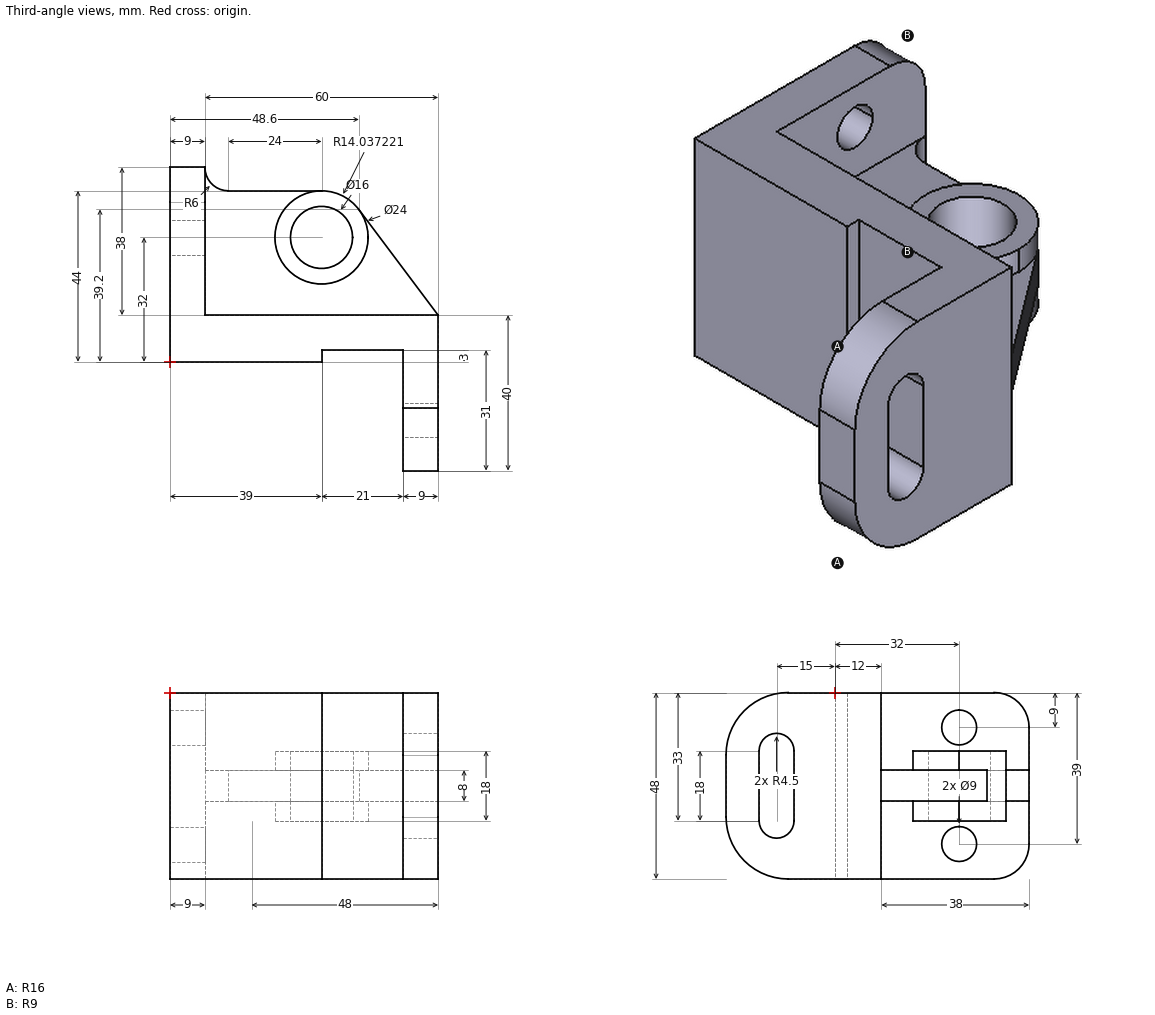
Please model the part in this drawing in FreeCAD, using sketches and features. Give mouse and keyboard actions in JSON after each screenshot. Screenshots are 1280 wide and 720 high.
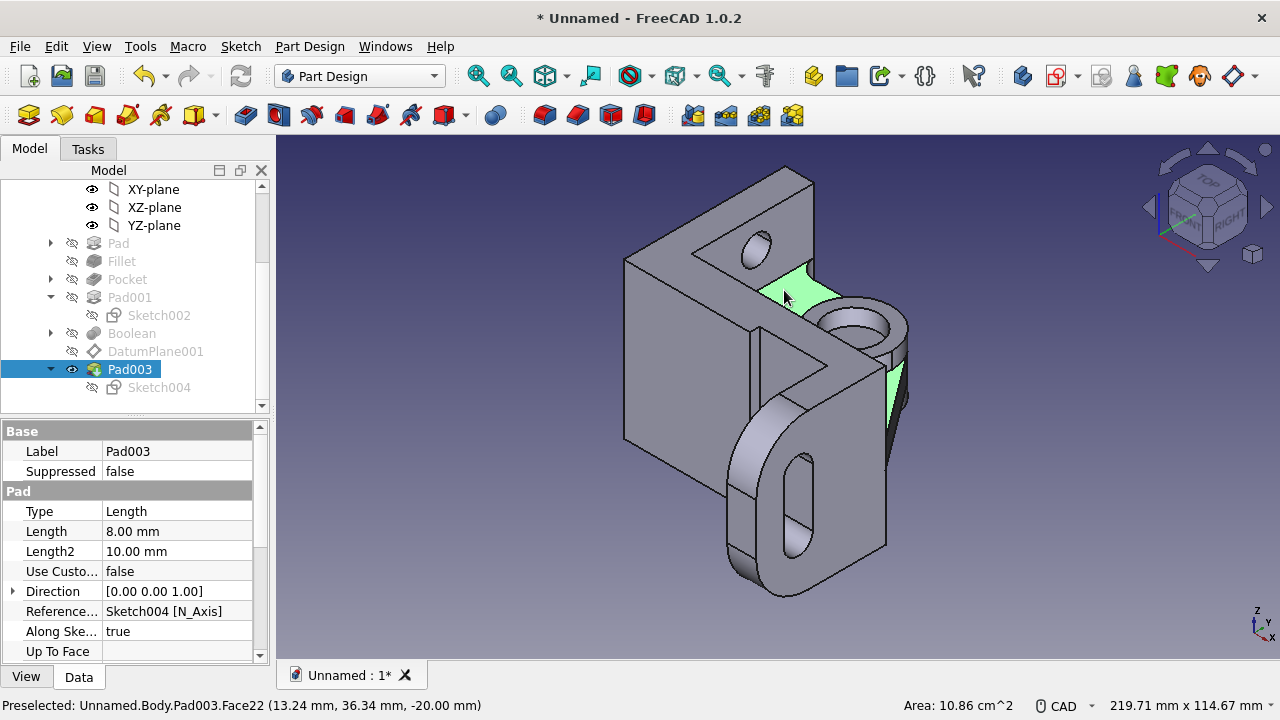
{"action": "left_click", "coordinate": [1056, 76]}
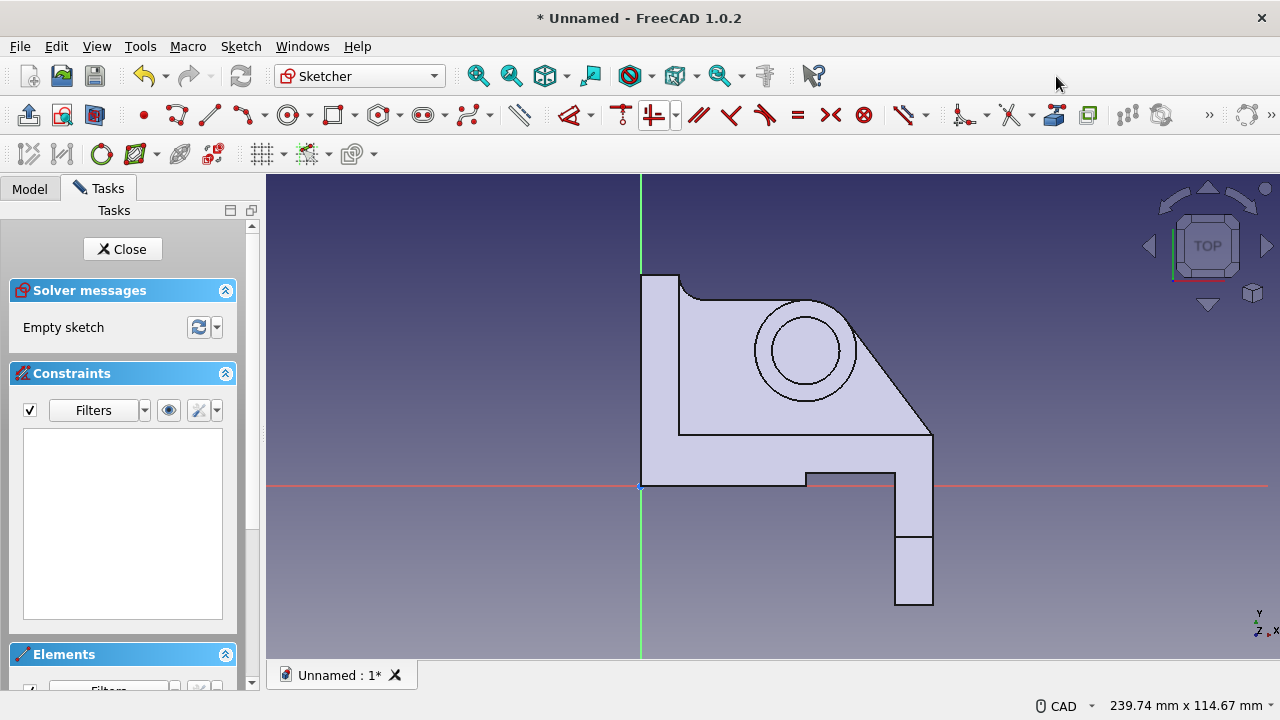
{"action": "left_click", "coordinate": [95, 116]}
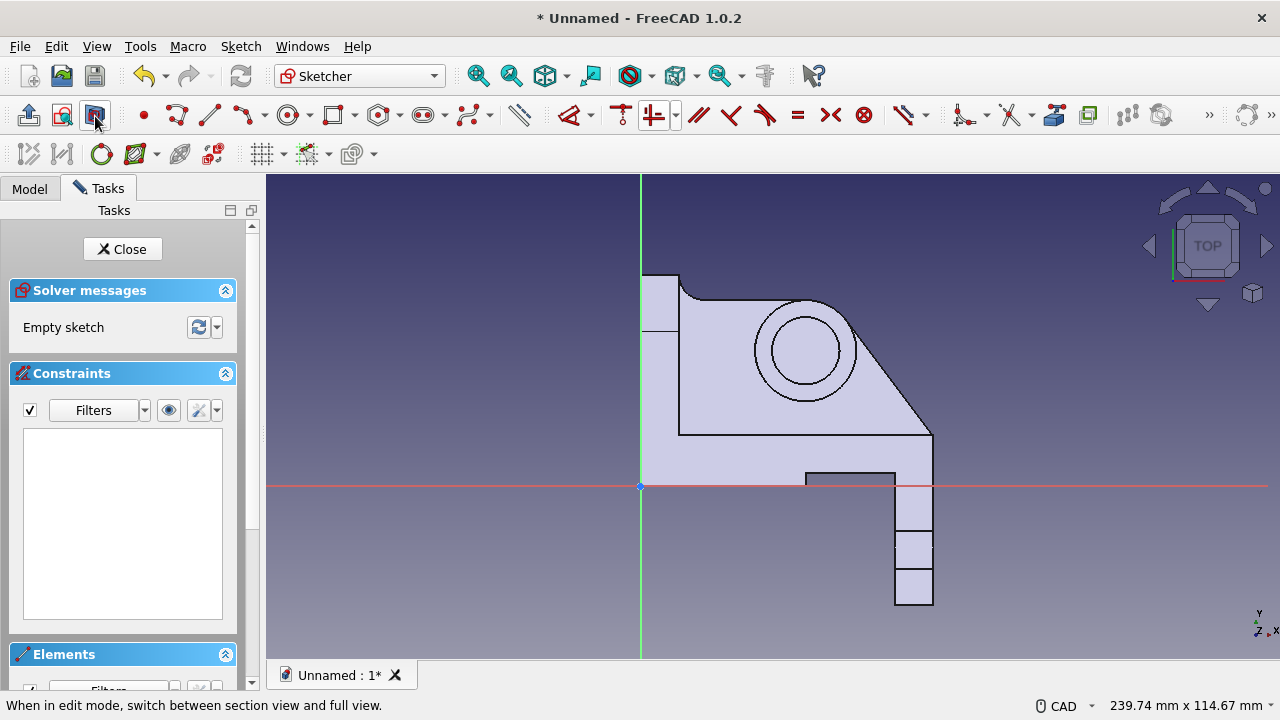
{"action": "scroll", "coordinate": [839, 329], "scroll_direction": "up", "scroll_amount": 7}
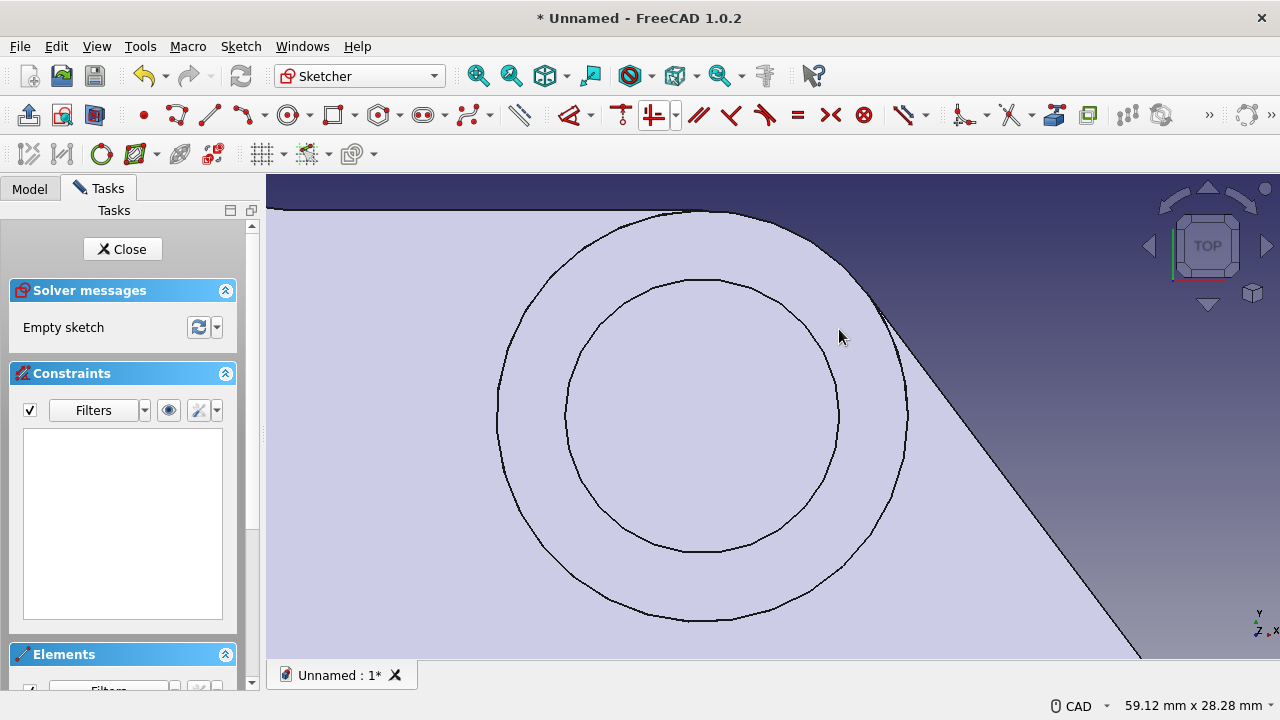
{"action": "key", "text": "g c"}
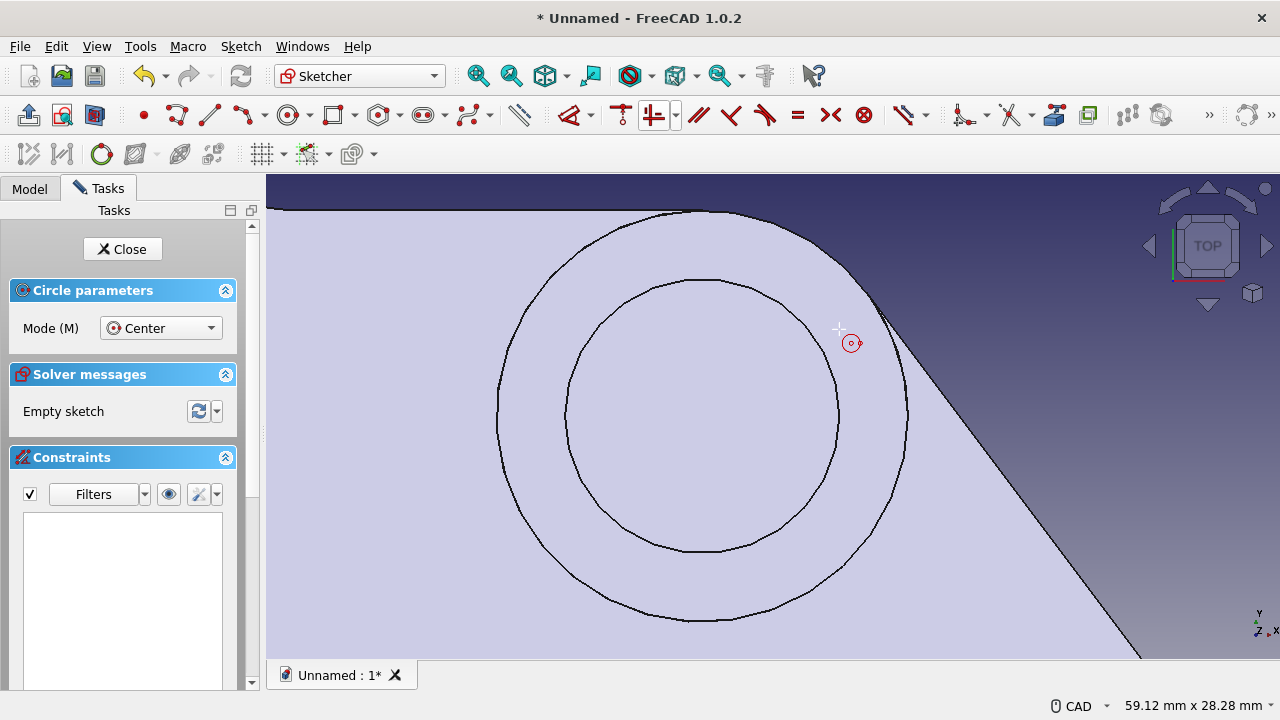
{"action": "left_click", "coordinate": [702, 416]}
{"action": "left_click", "coordinate": [799, 319]}
{"action": "key", "text": "Escape"}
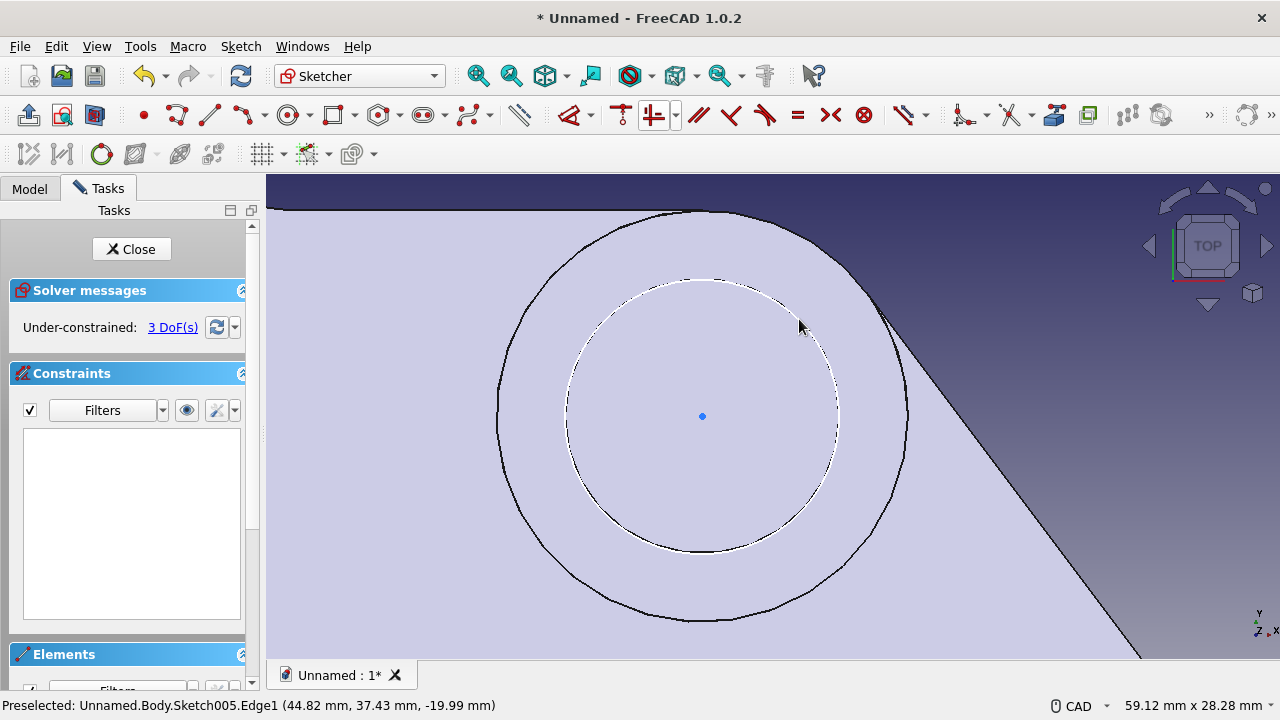
{"action": "key", "text": "d"}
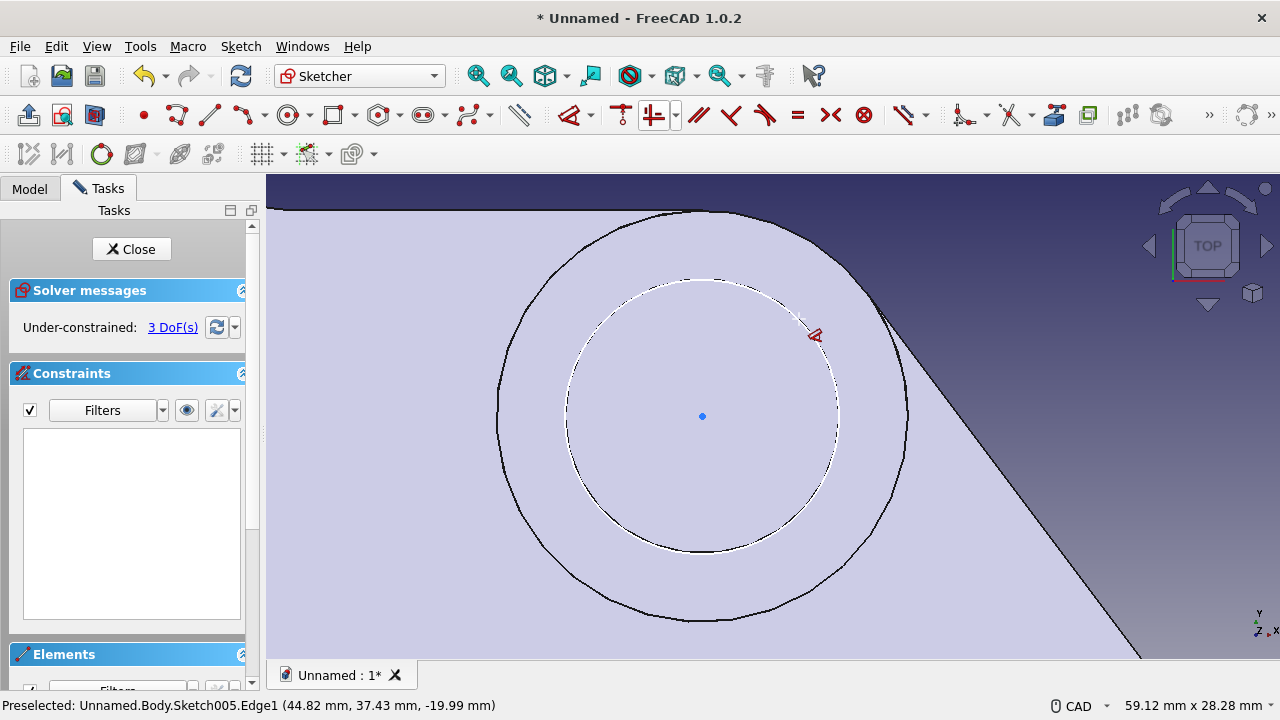
{"action": "left_click", "coordinate": [799, 320]}
{"action": "left_click", "coordinate": [822, 297]}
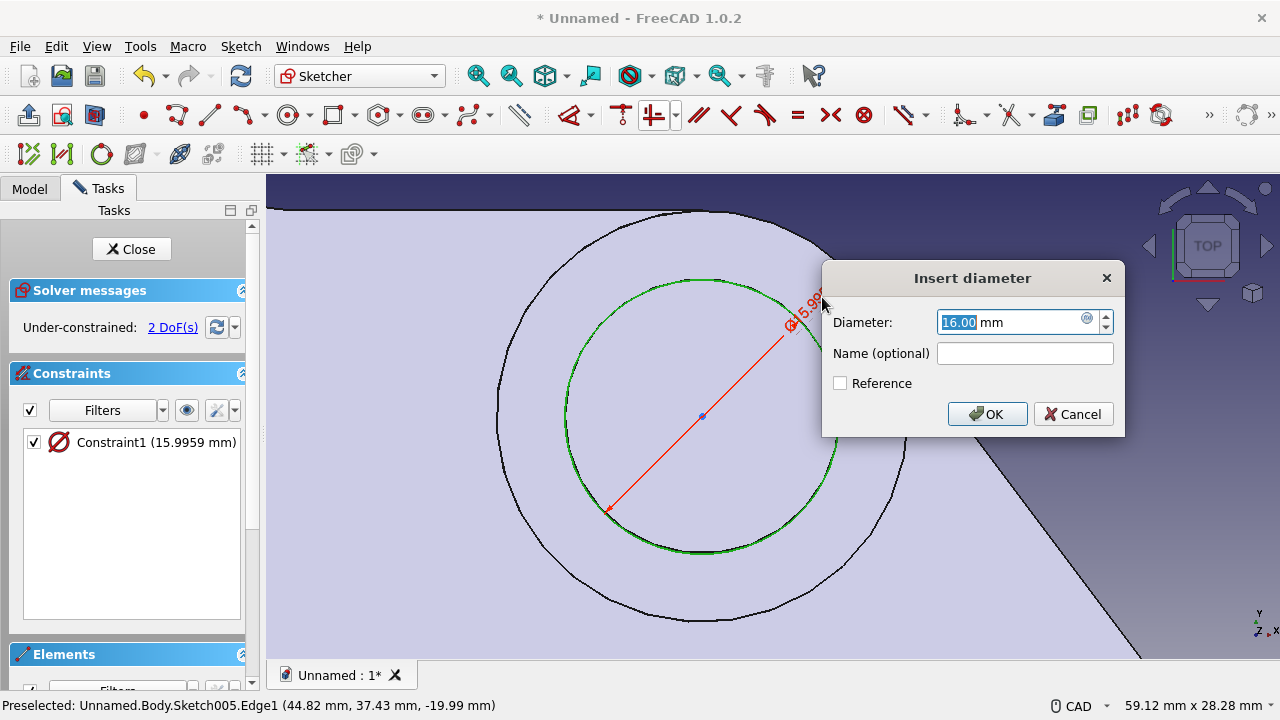
{"action": "type", "text": "16"}
{"action": "key", "text": "Return"}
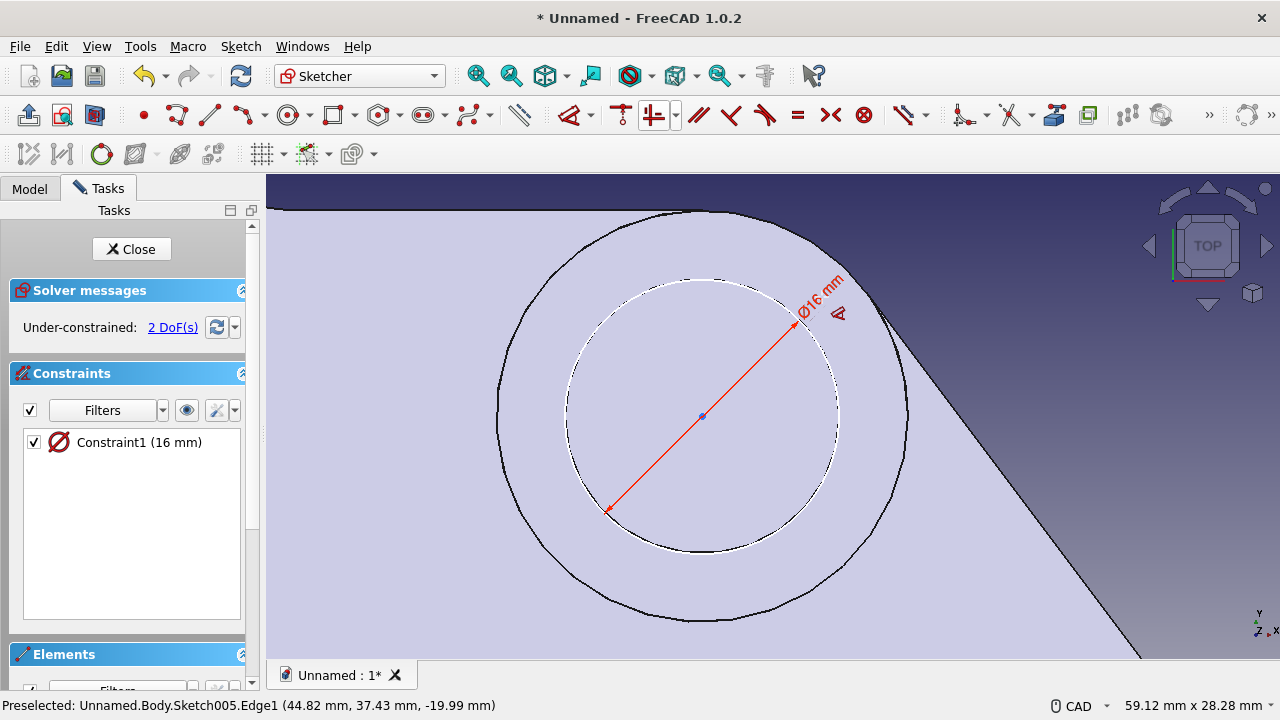
{"action": "left_click", "coordinate": [702, 417]}
{"action": "left_click", "coordinate": [498, 383]}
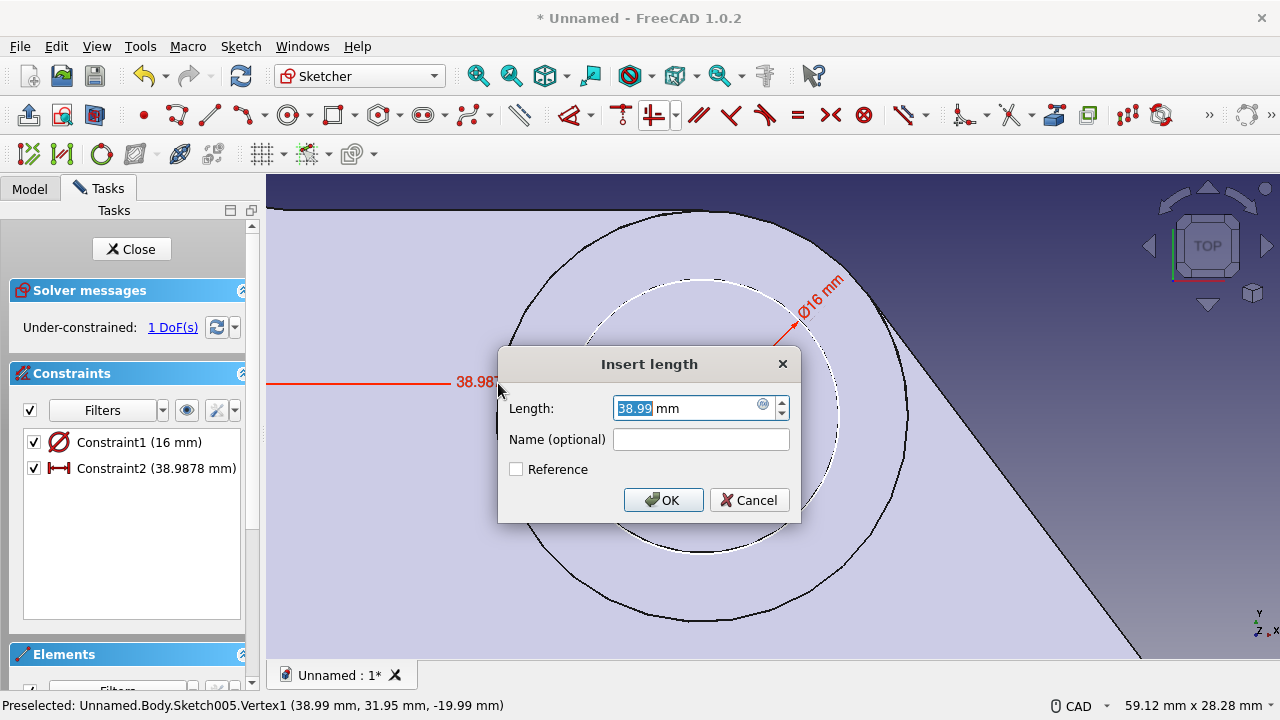
{"action": "type", "text": "39"}
{"action": "key", "text": "Return"}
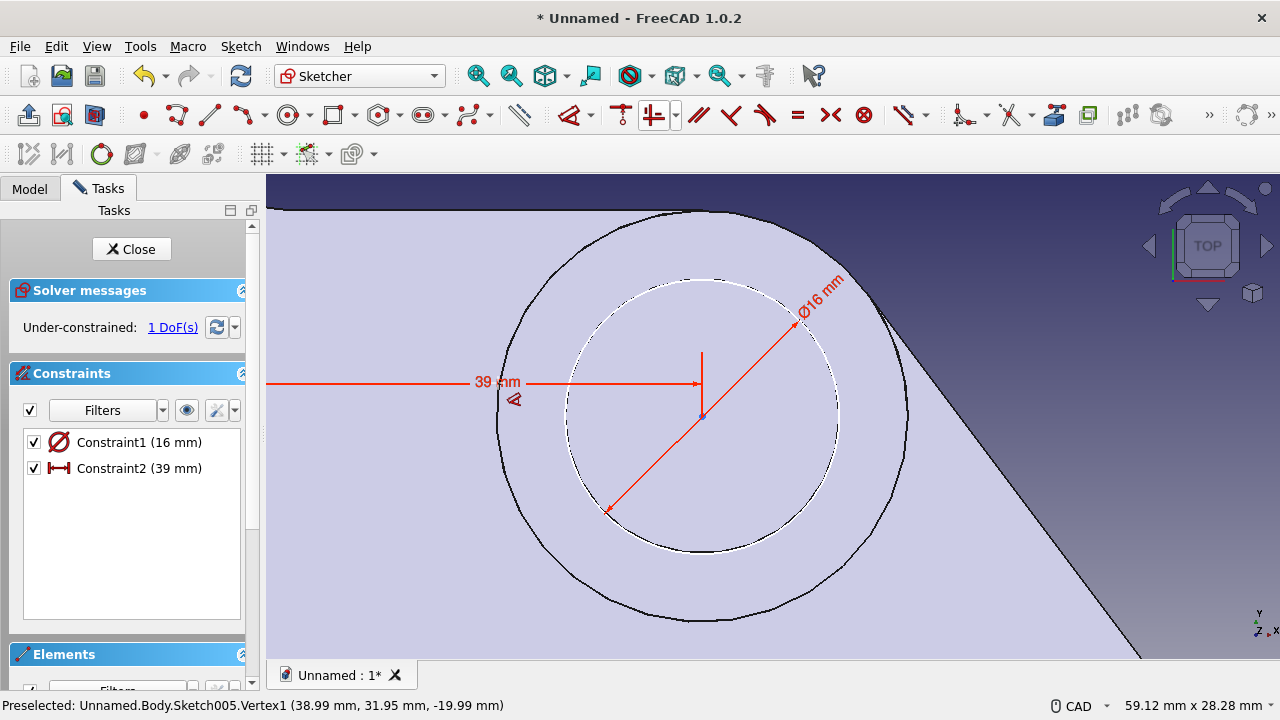
{"action": "left_click", "coordinate": [702, 417]}
{"action": "left_click", "coordinate": [736, 524]}